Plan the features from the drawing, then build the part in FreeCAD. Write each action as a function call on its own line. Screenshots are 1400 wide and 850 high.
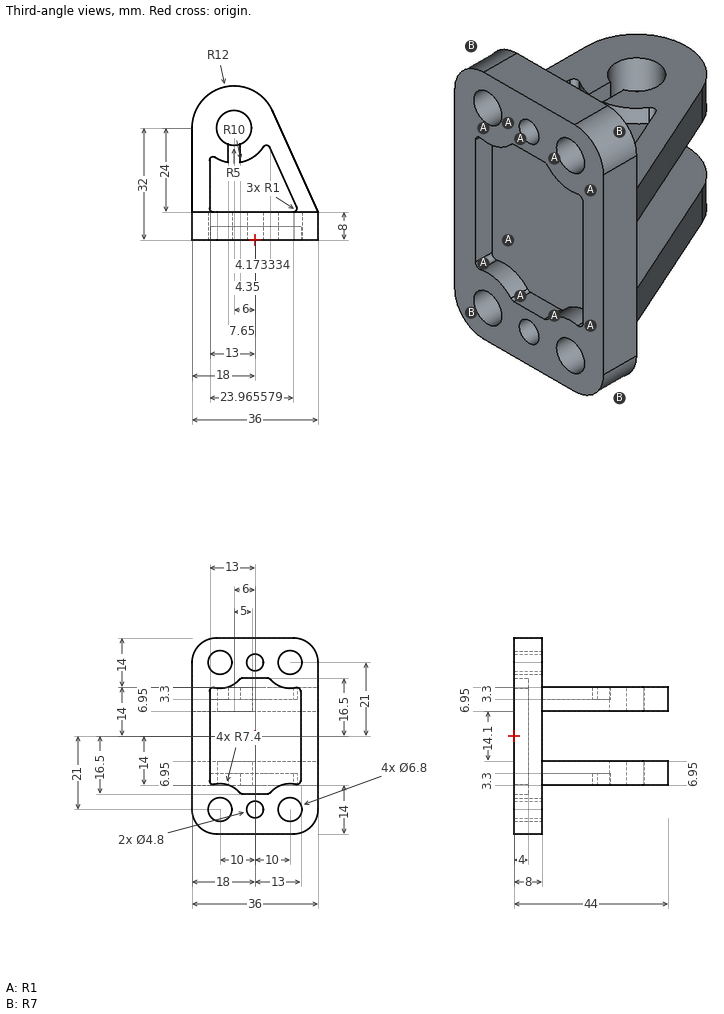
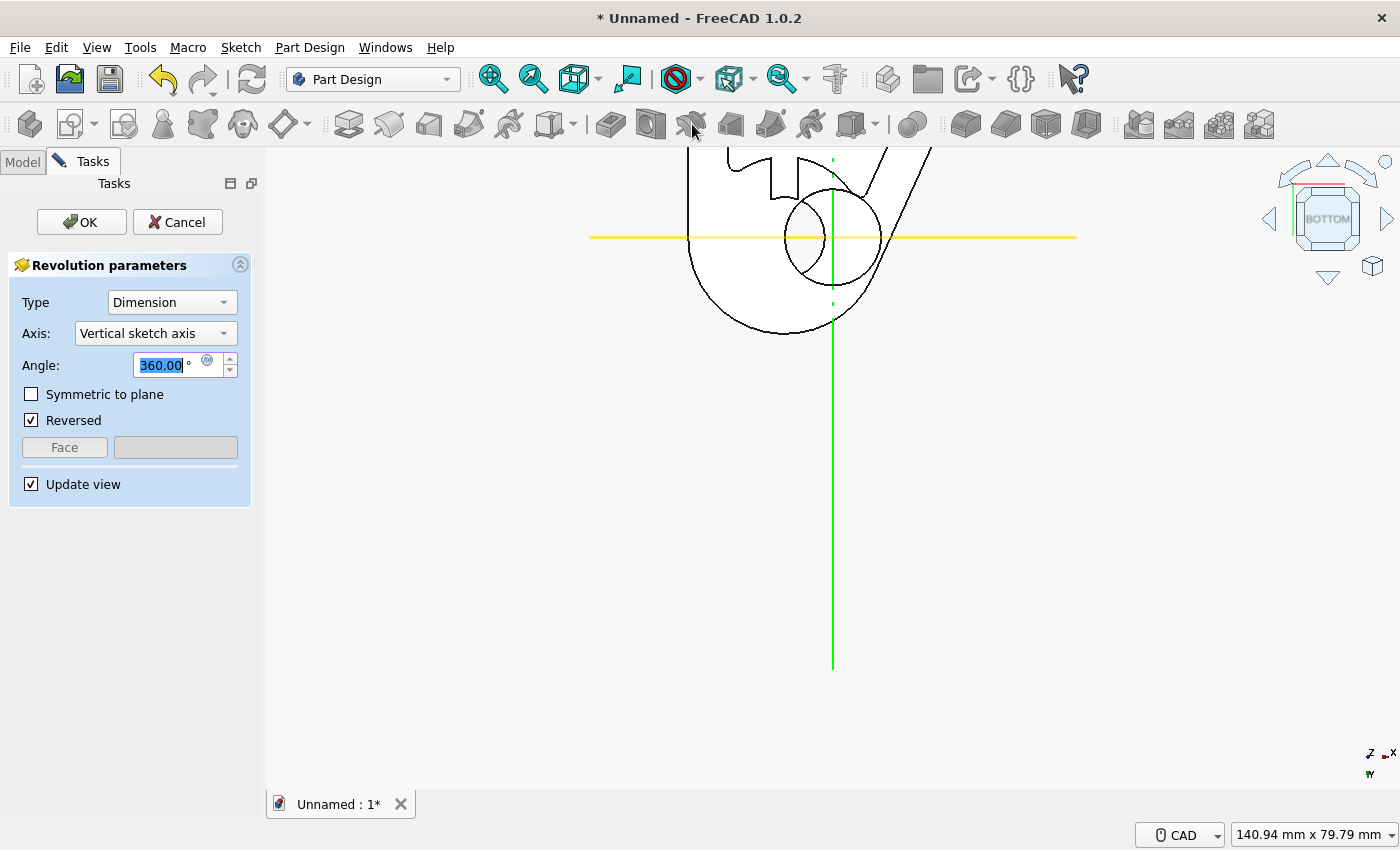
click(156, 334)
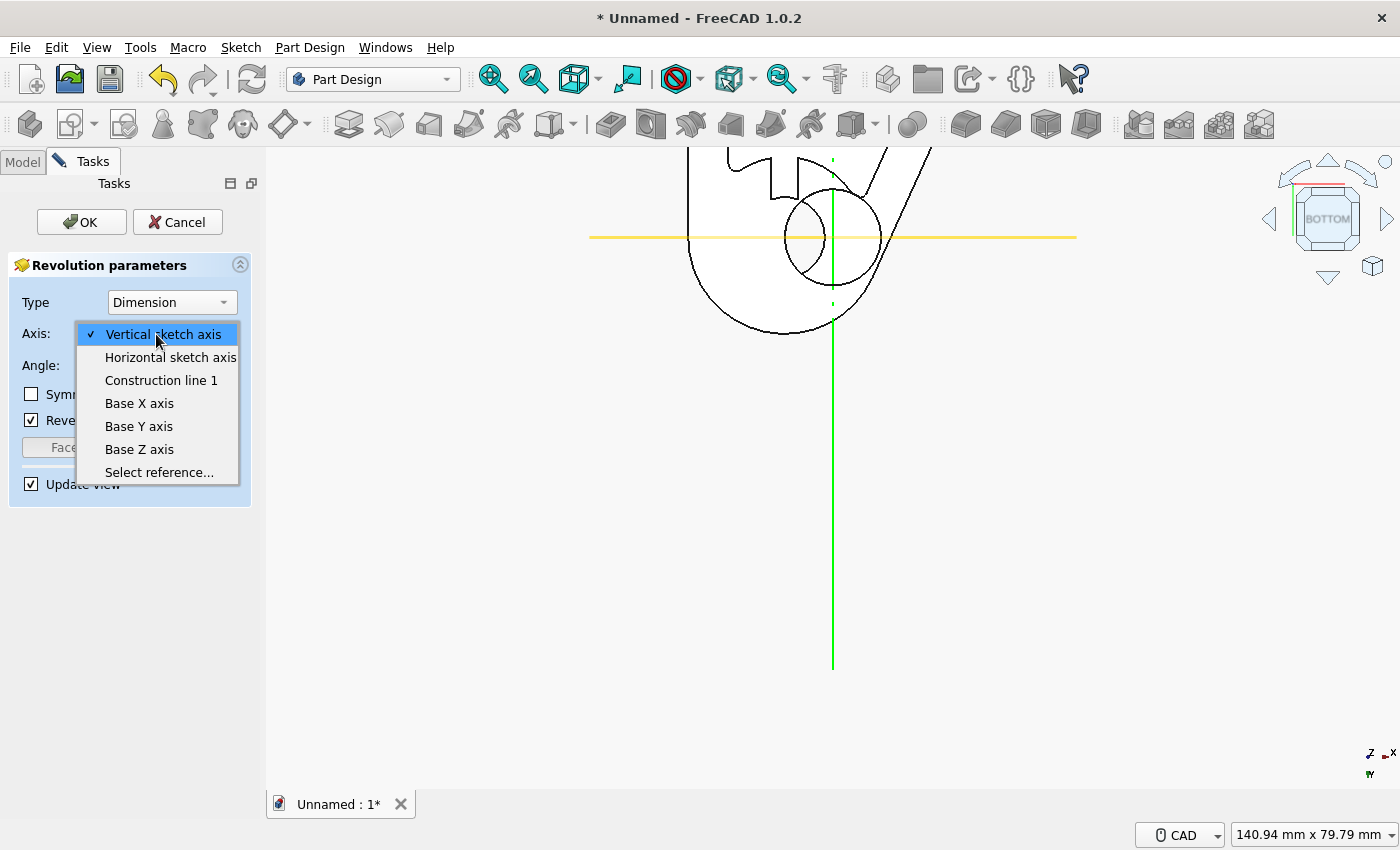
click(156, 380)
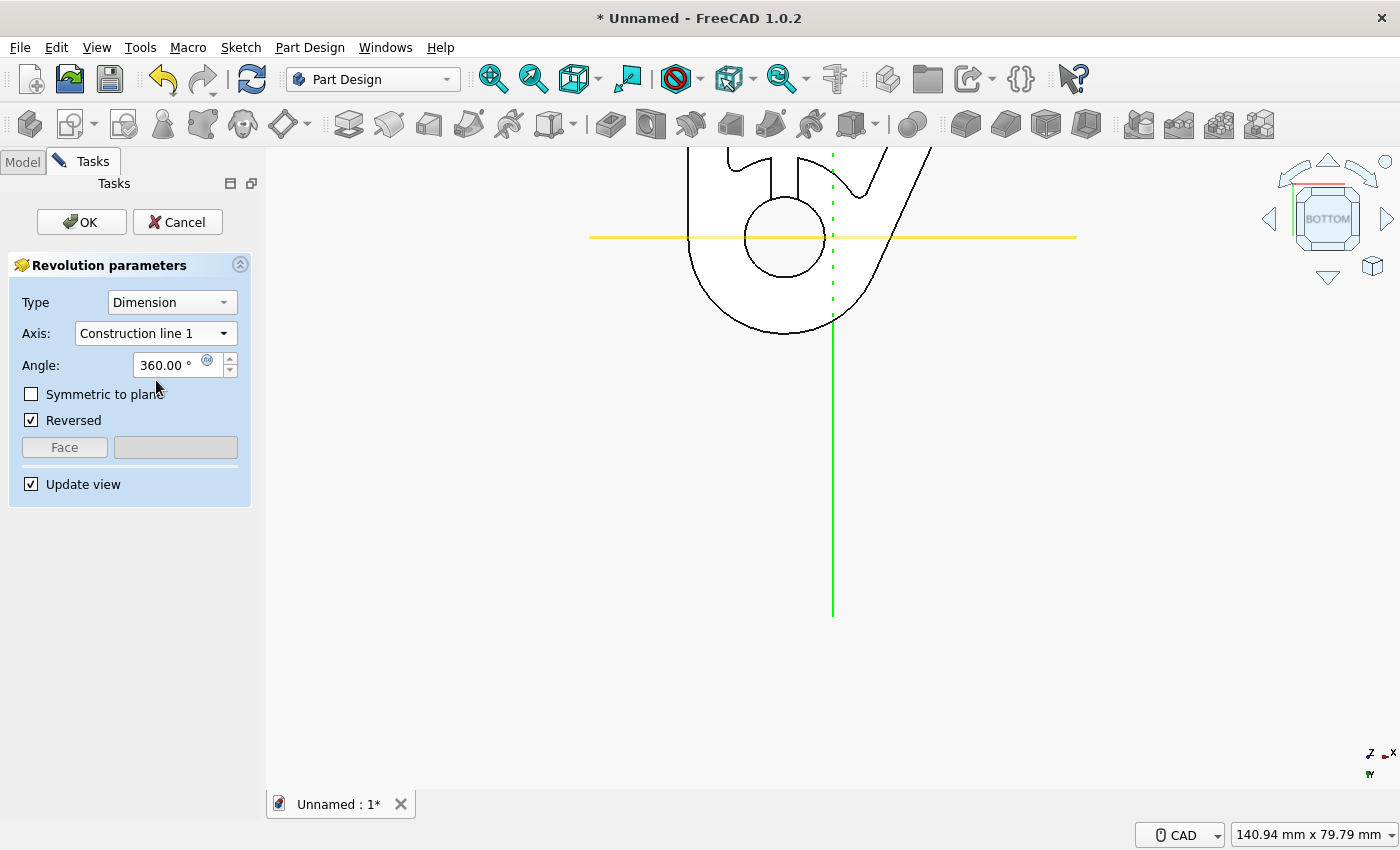
click(82, 222)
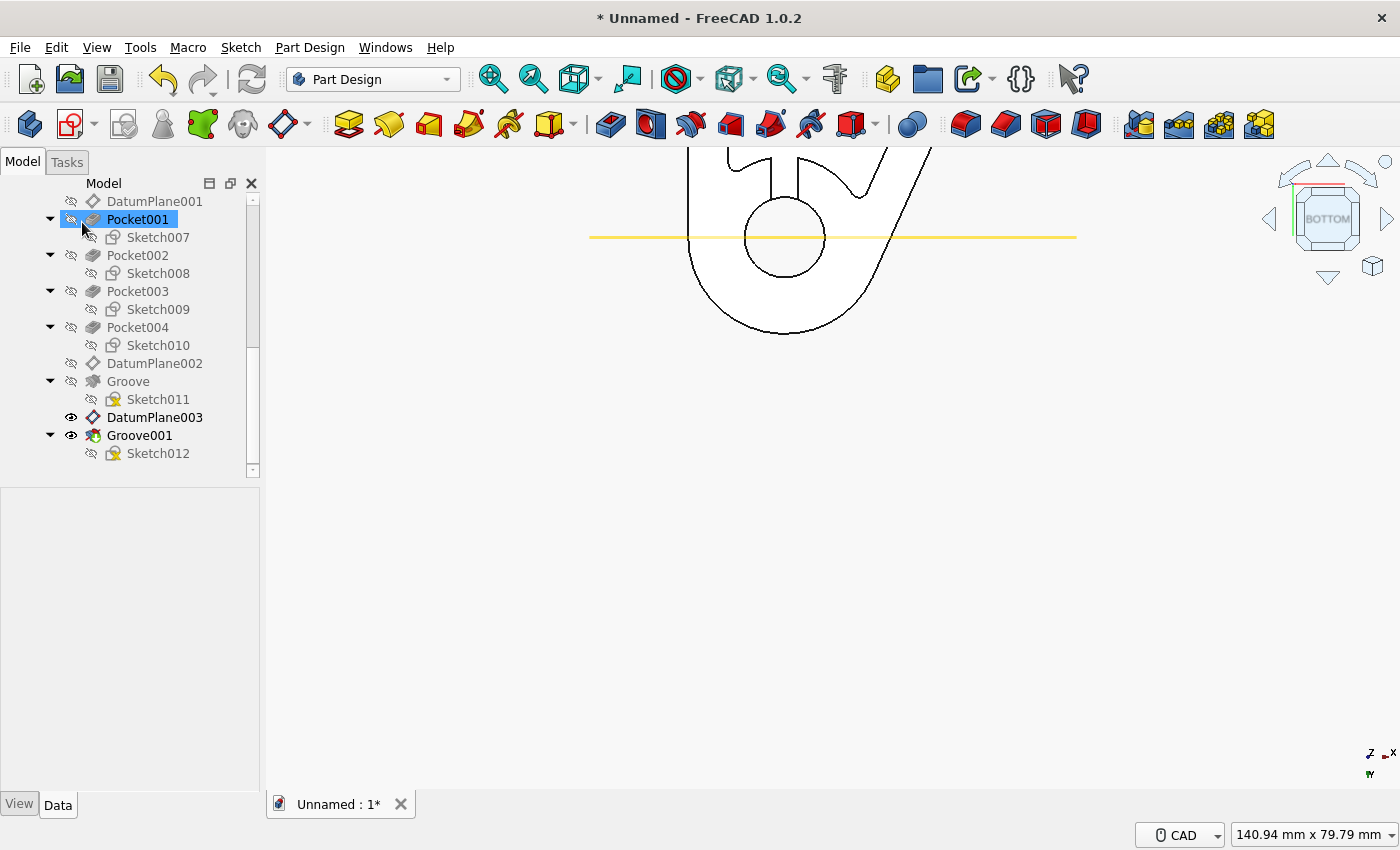
click(116, 417)
key(space)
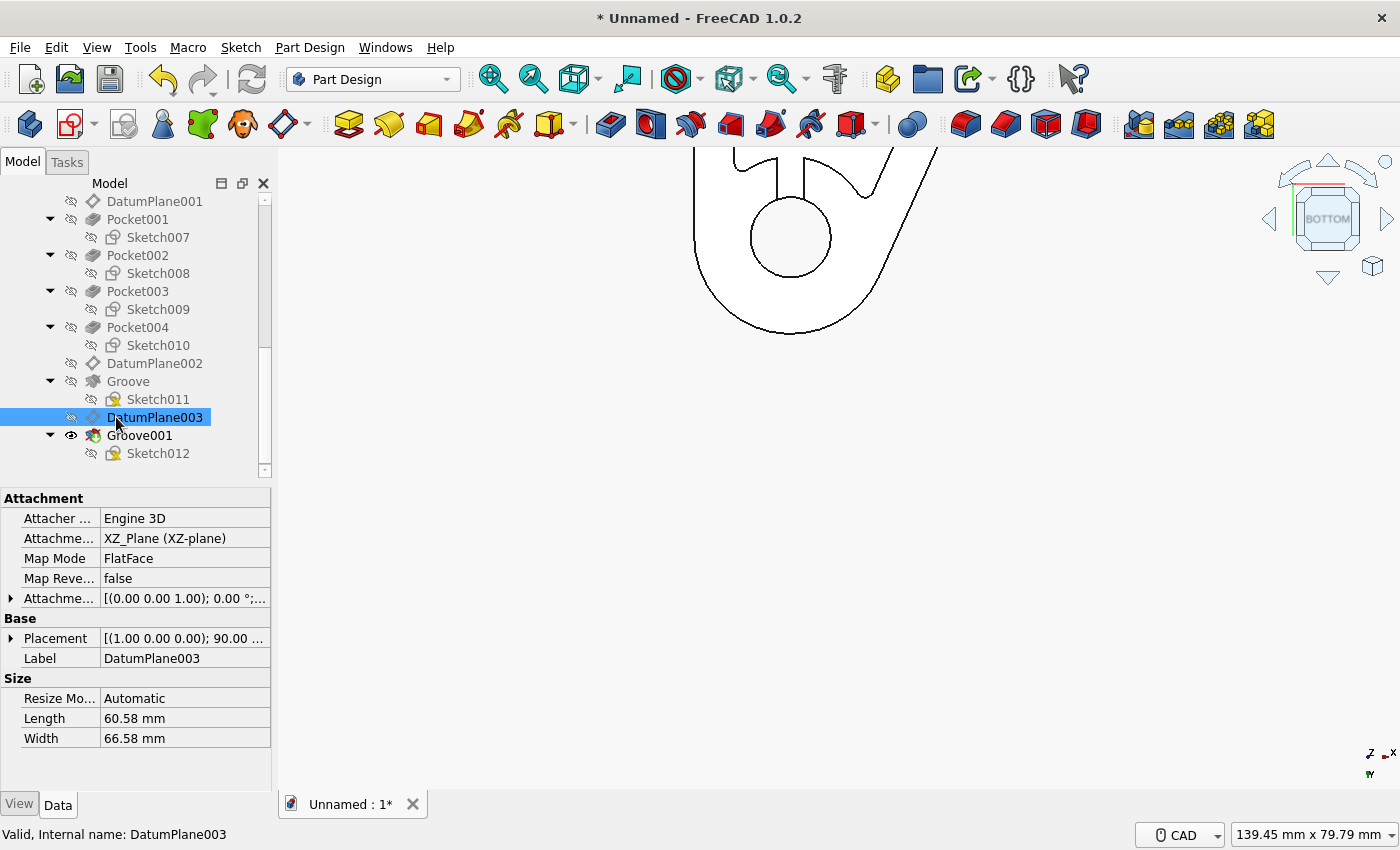
key(v)
key(f)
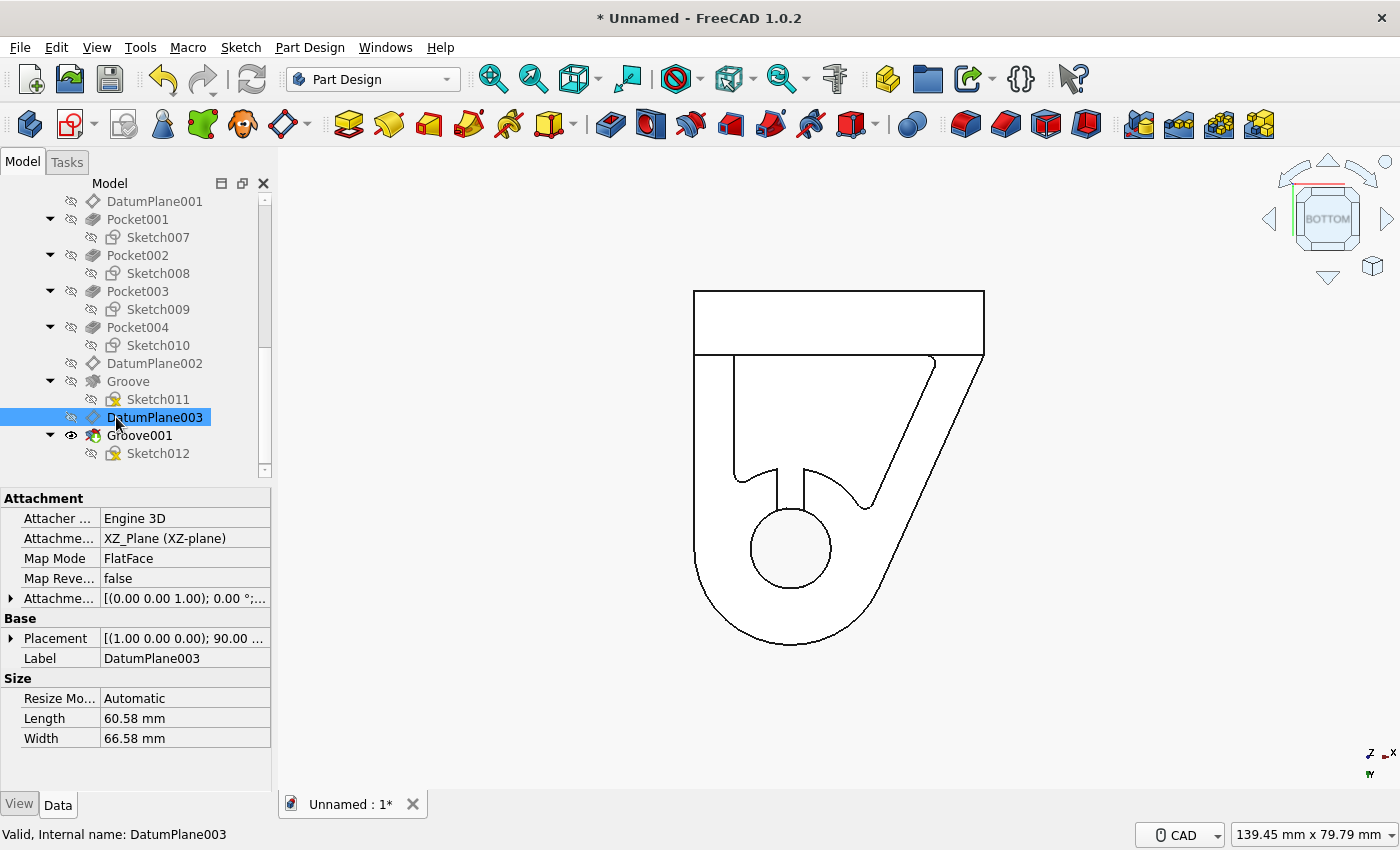
click(318, 749)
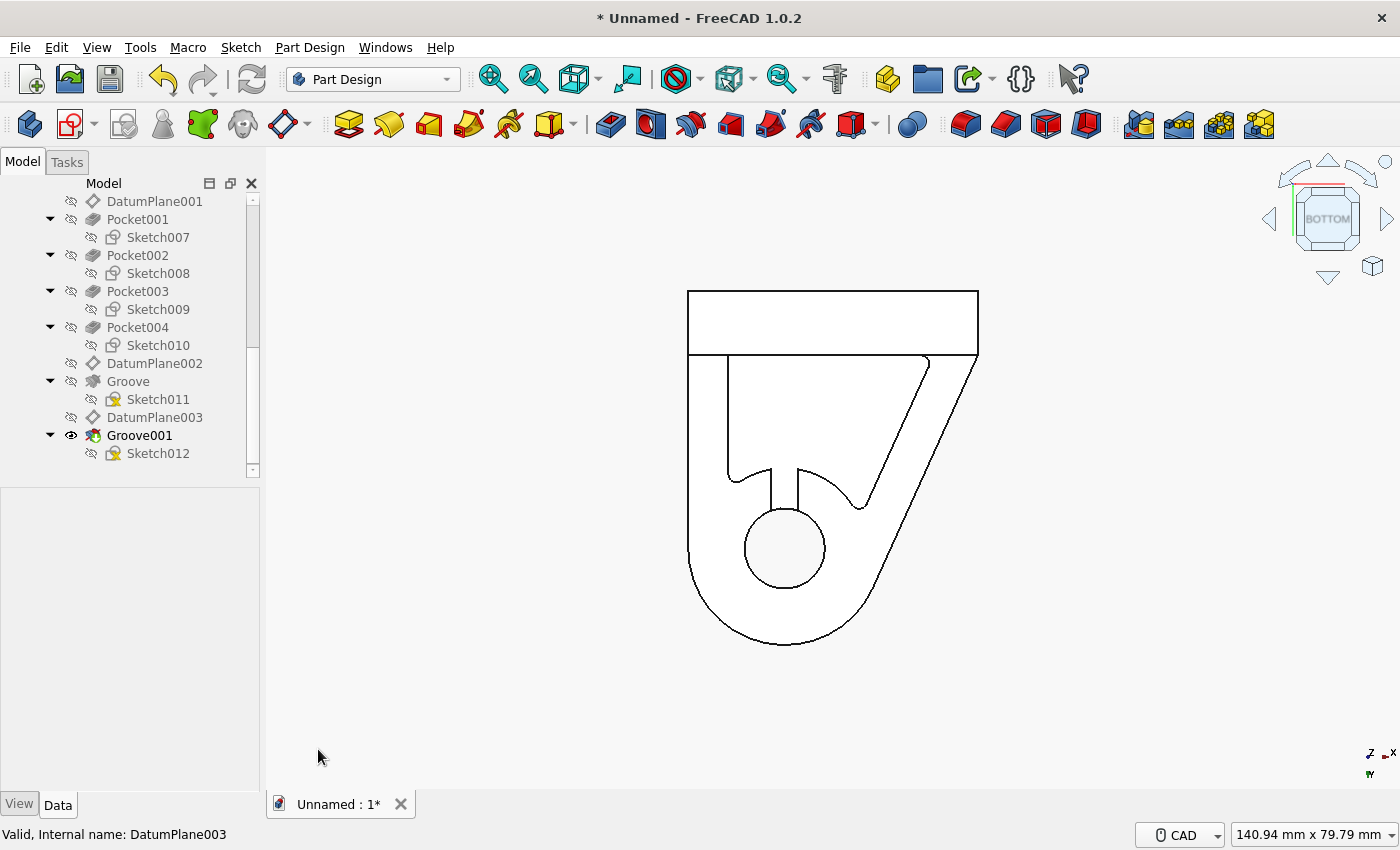
click(70, 124)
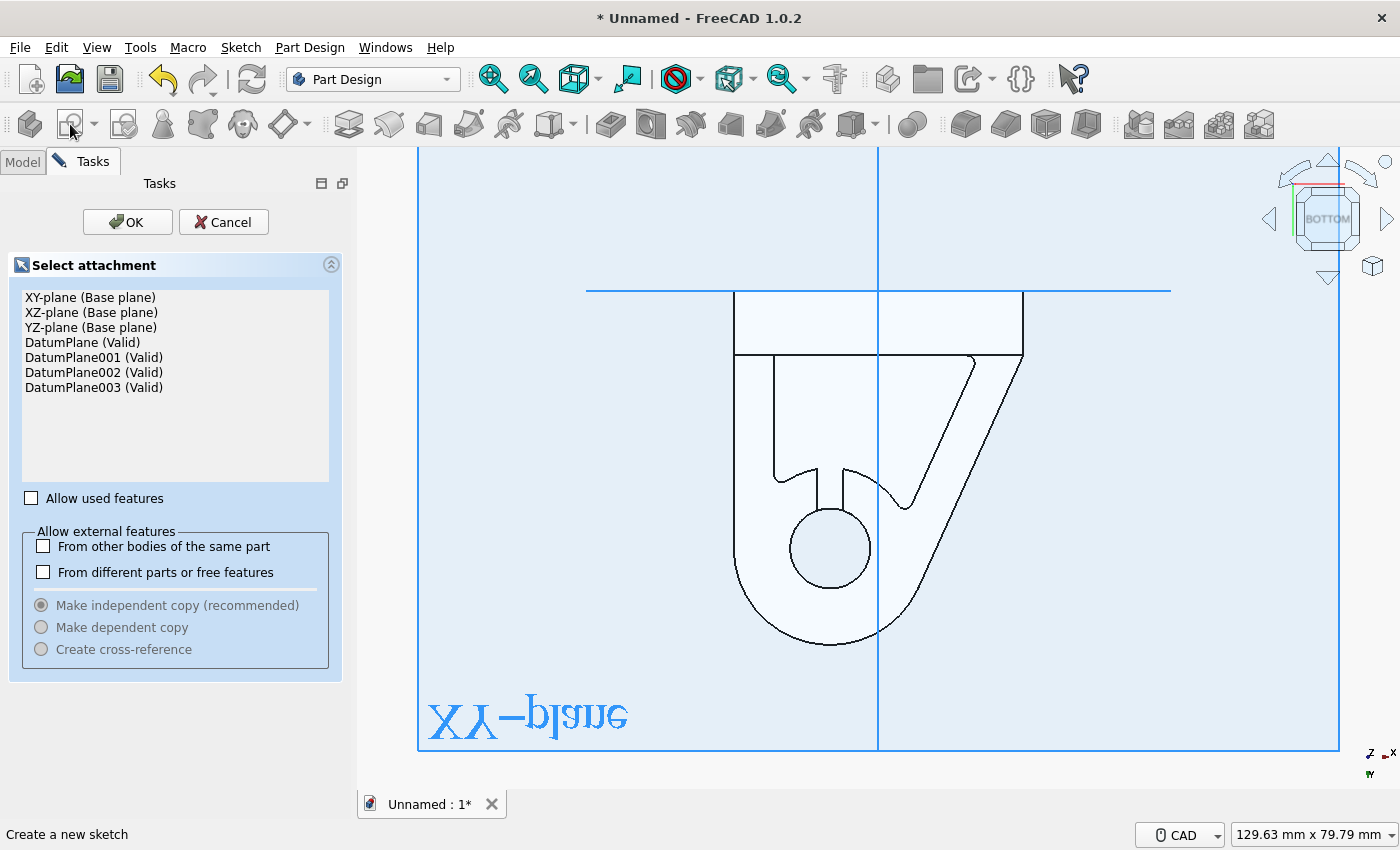
click(82, 312)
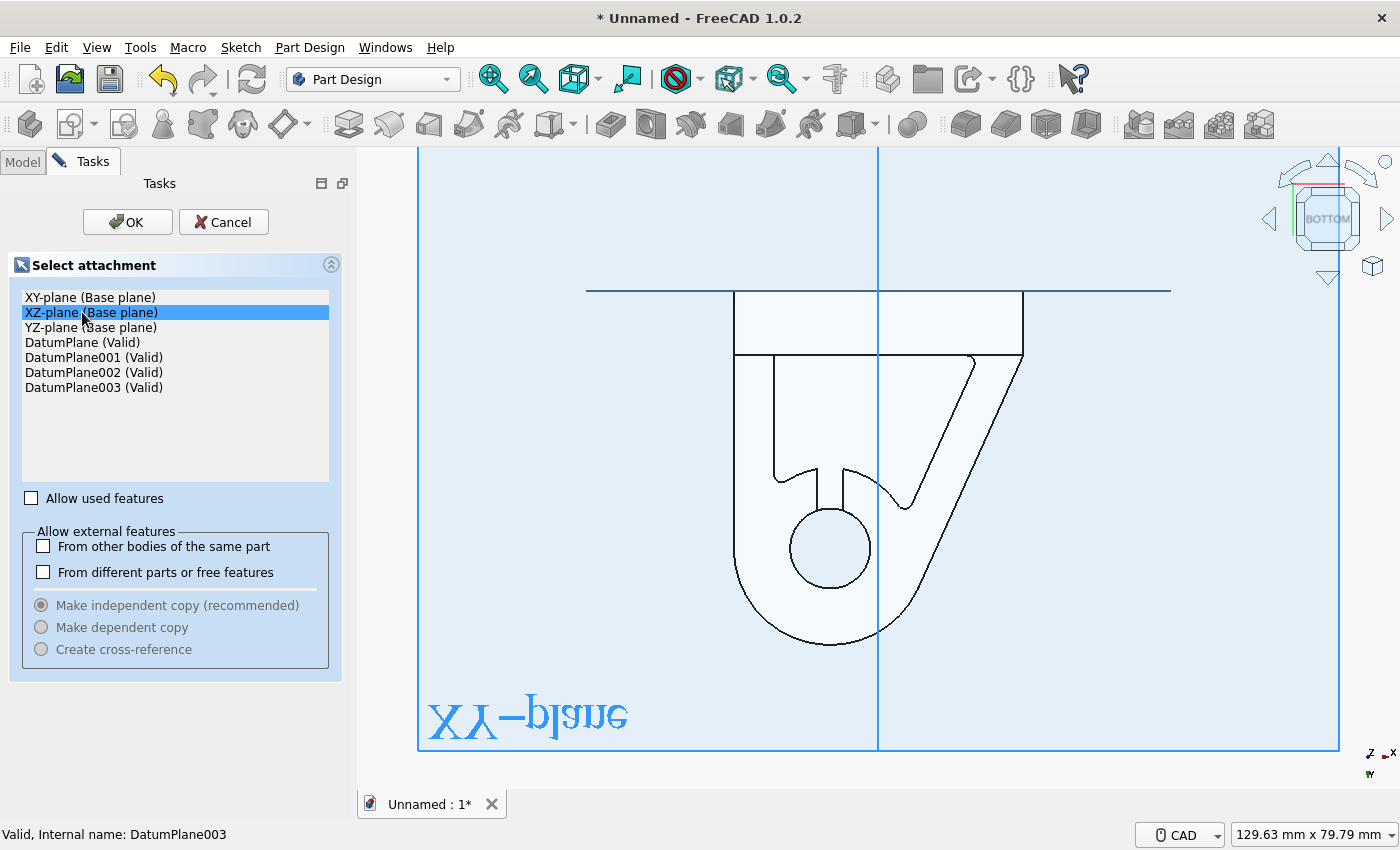
click(128, 222)